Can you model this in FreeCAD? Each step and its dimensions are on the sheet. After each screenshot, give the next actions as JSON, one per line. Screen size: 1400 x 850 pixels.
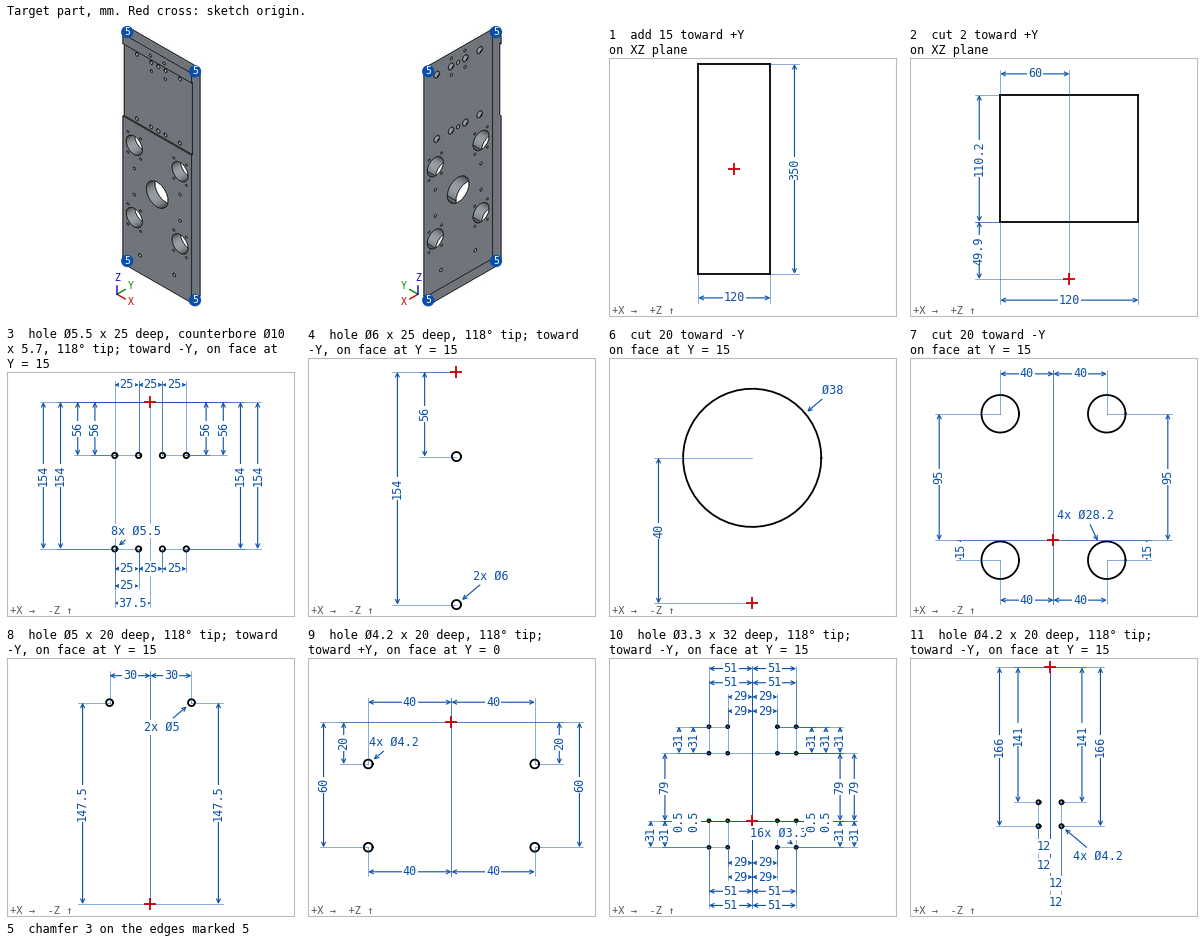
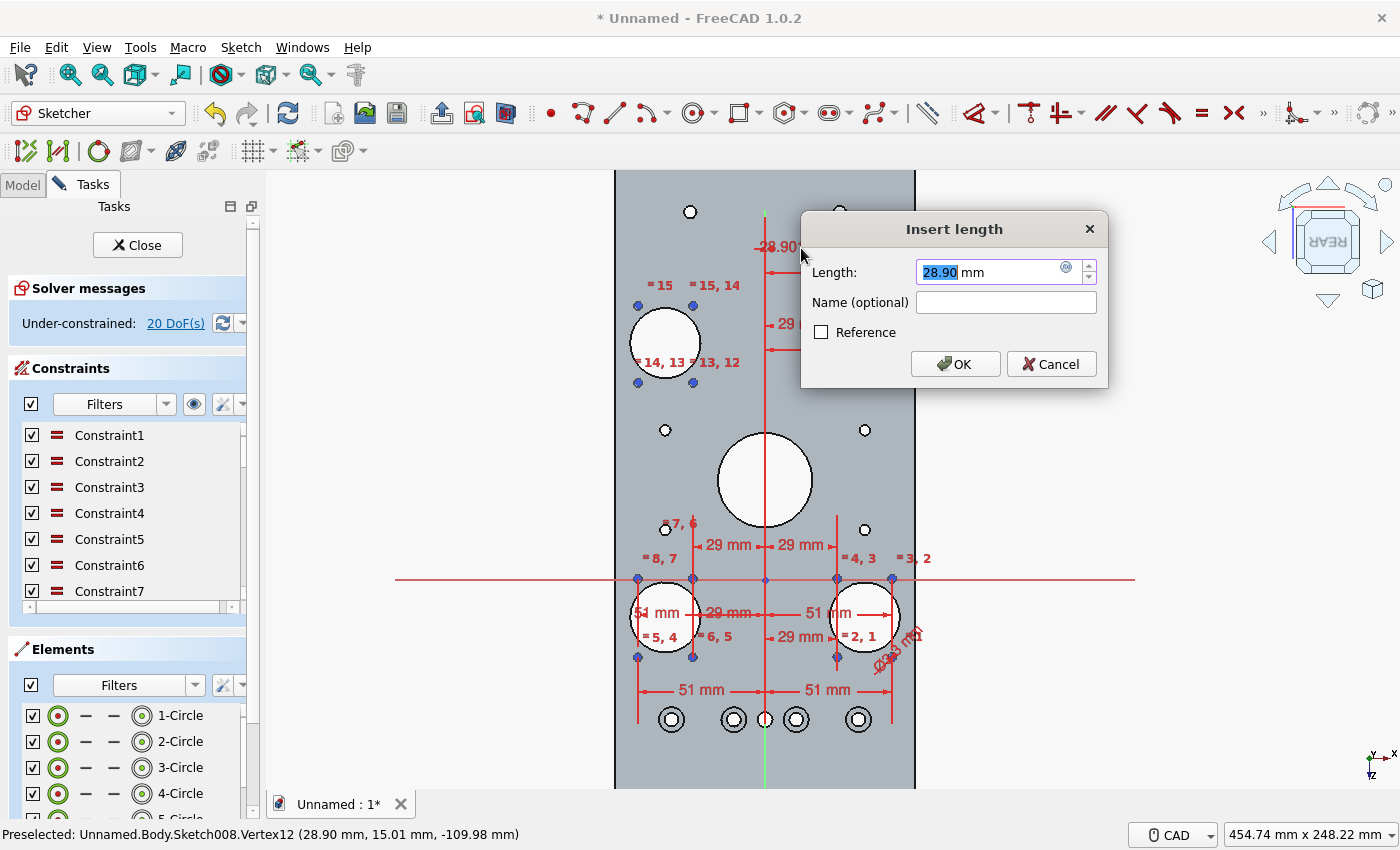
{"action": "type", "text": "29"}
{"action": "key", "text": "Return"}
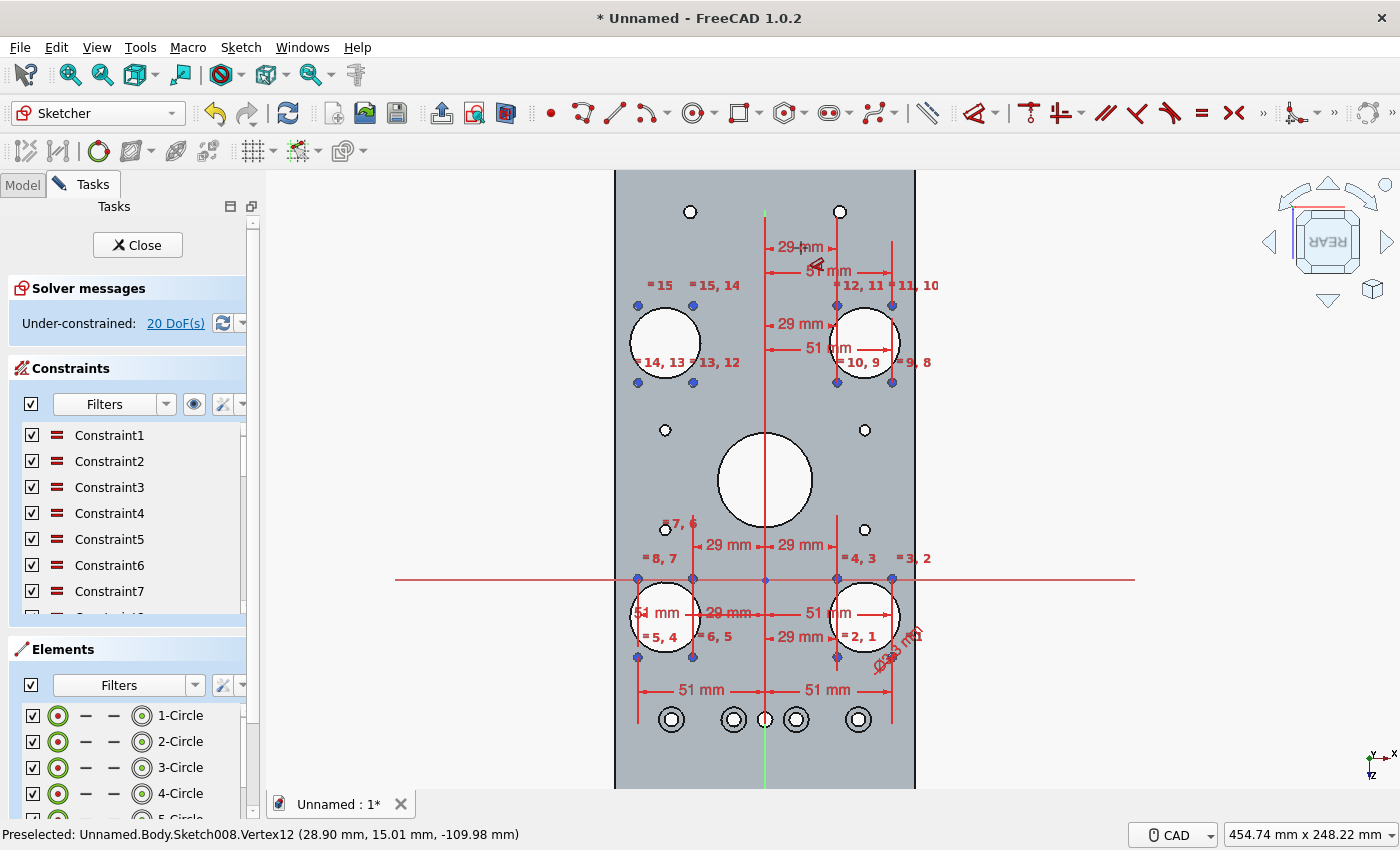
{"action": "left_click", "coordinate": [693, 383]}
{"action": "left_click", "coordinate": [729, 349]}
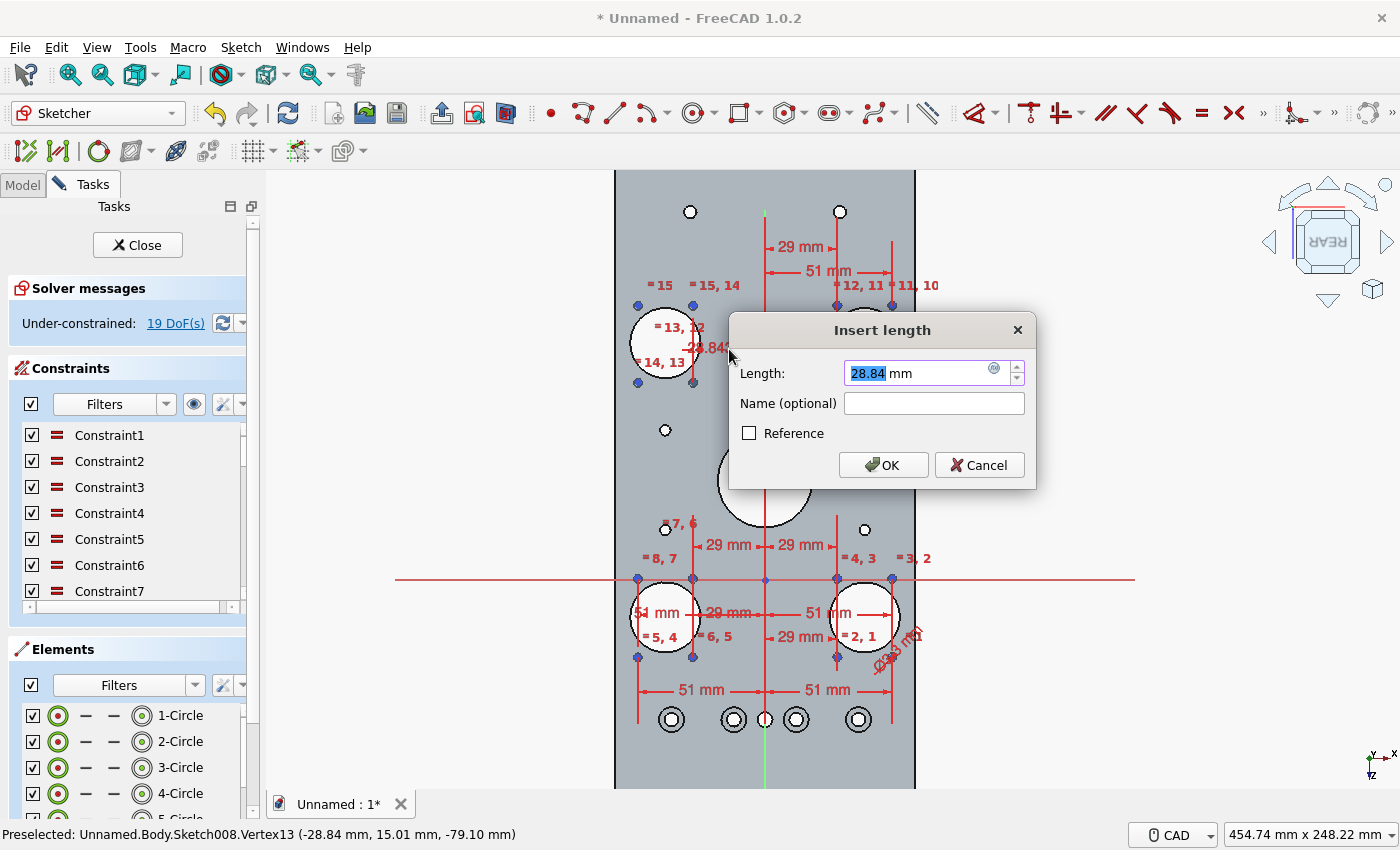
{"action": "type", "text": "29"}
{"action": "key", "text": "Return"}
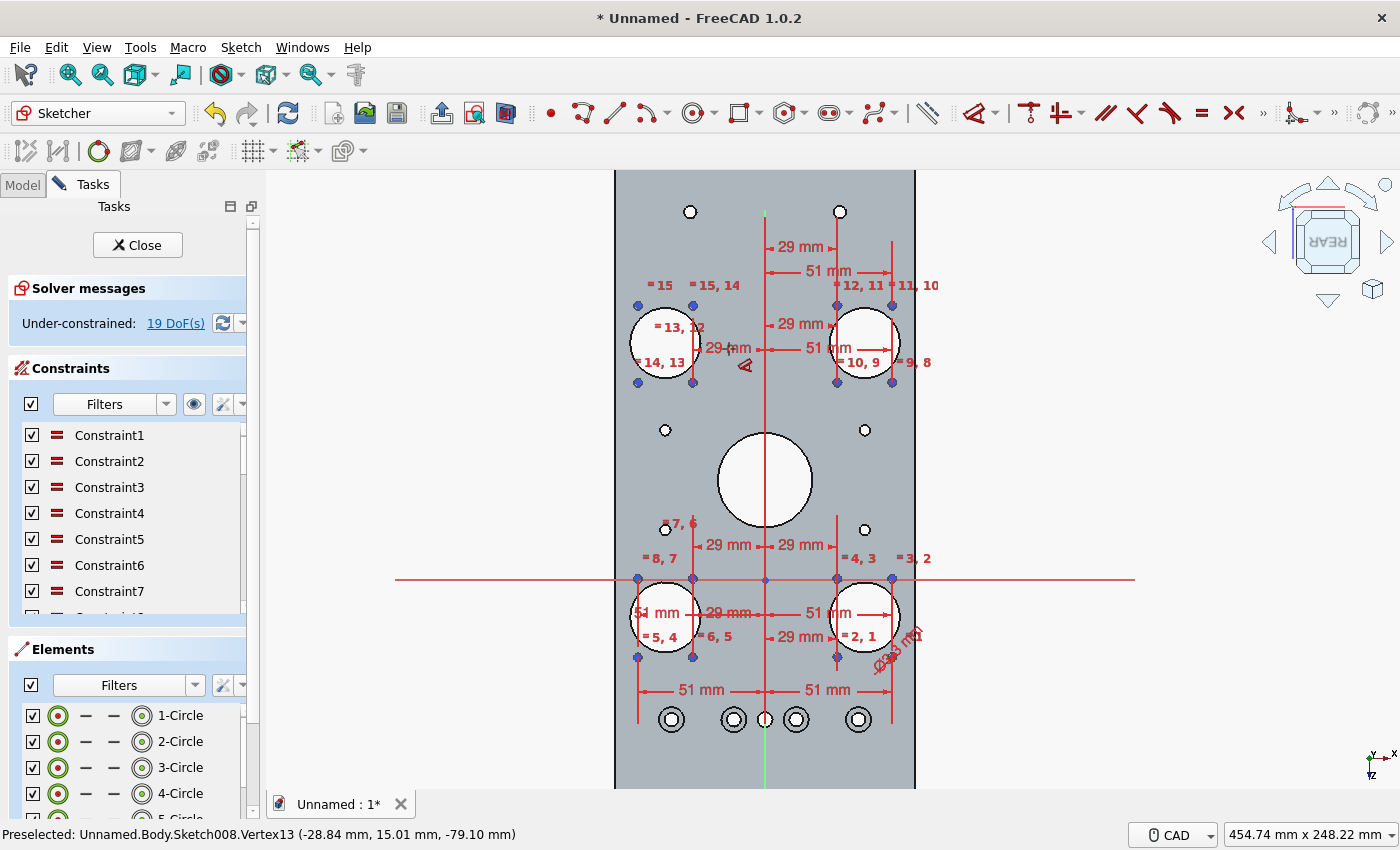
{"action": "left_click", "coordinate": [638, 383]}
{"action": "left_click", "coordinate": [657, 349]}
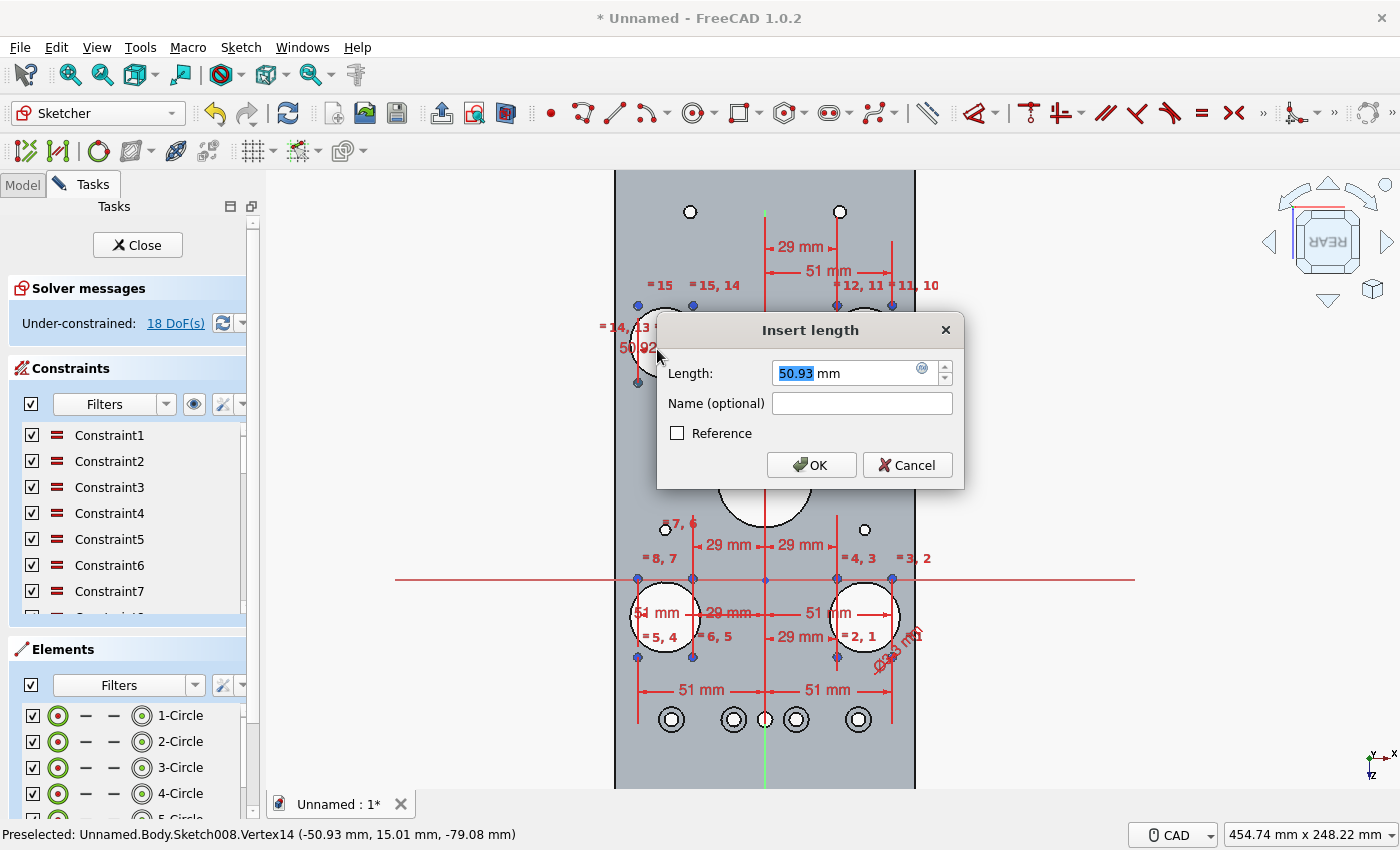
{"action": "type", "text": "51"}
{"action": "key", "text": "Return"}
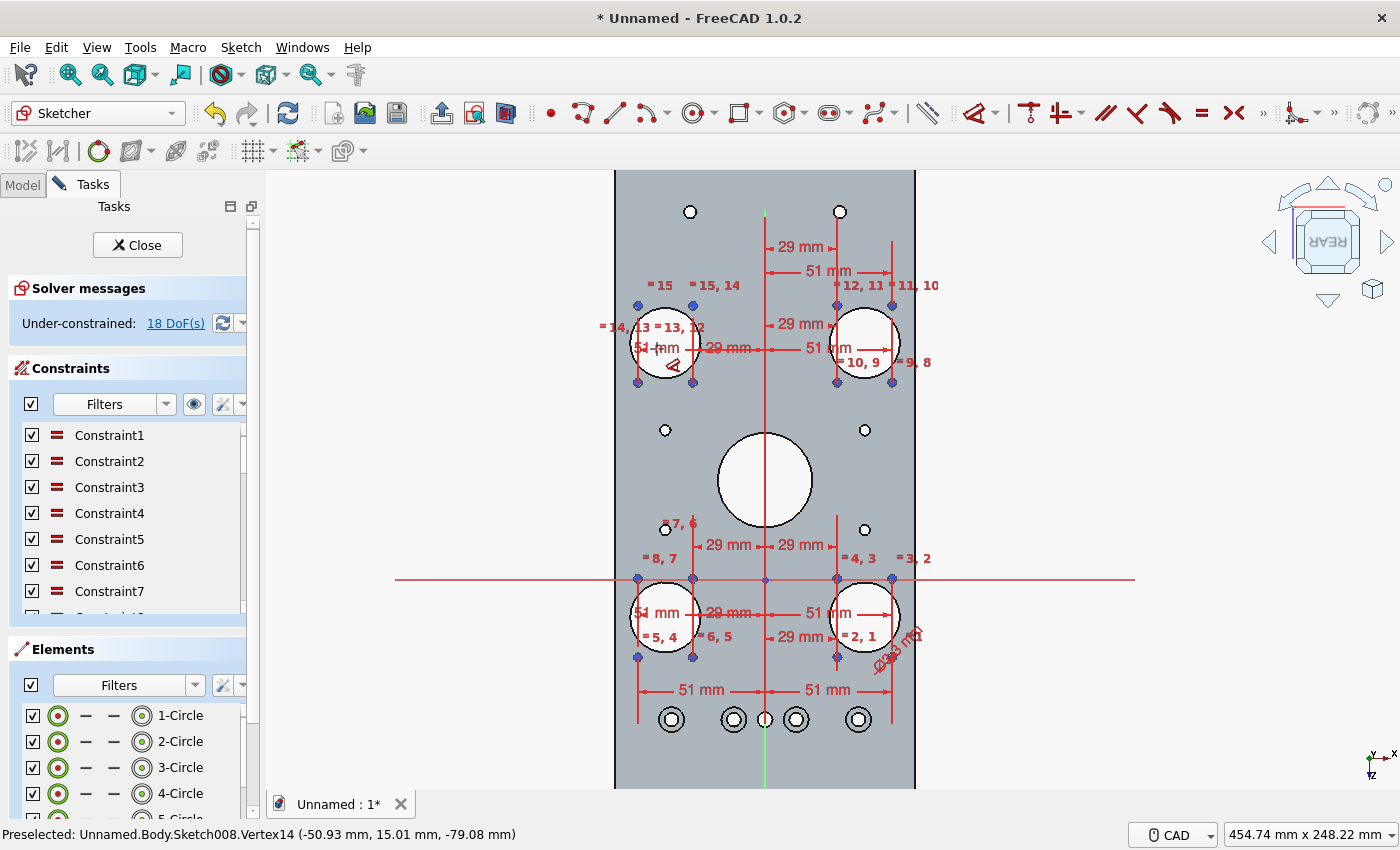
{"action": "left_click", "coordinate": [693, 306]}
{"action": "left_click", "coordinate": [729, 272]}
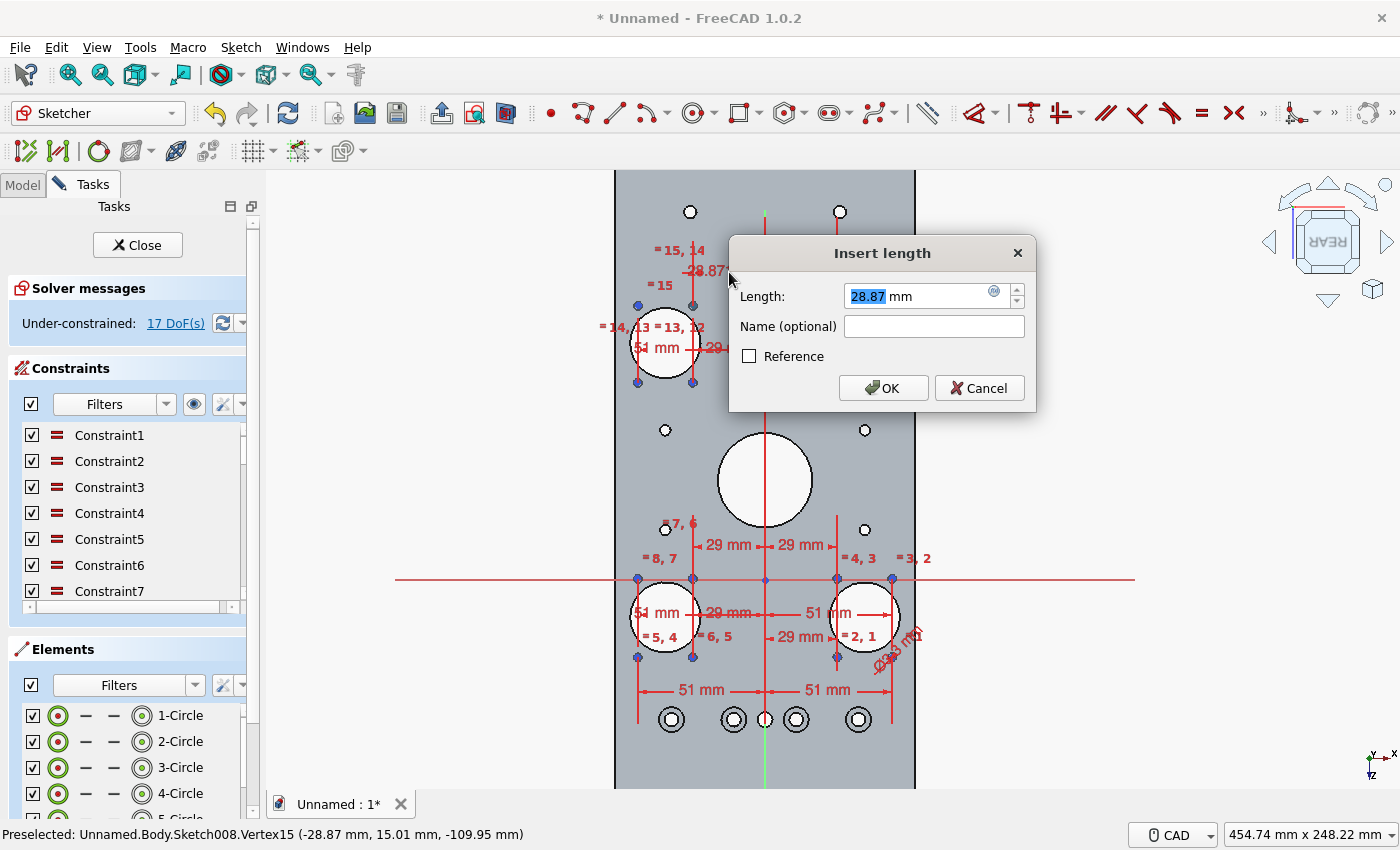
{"action": "type", "text": "29"}
{"action": "key", "text": "Return"}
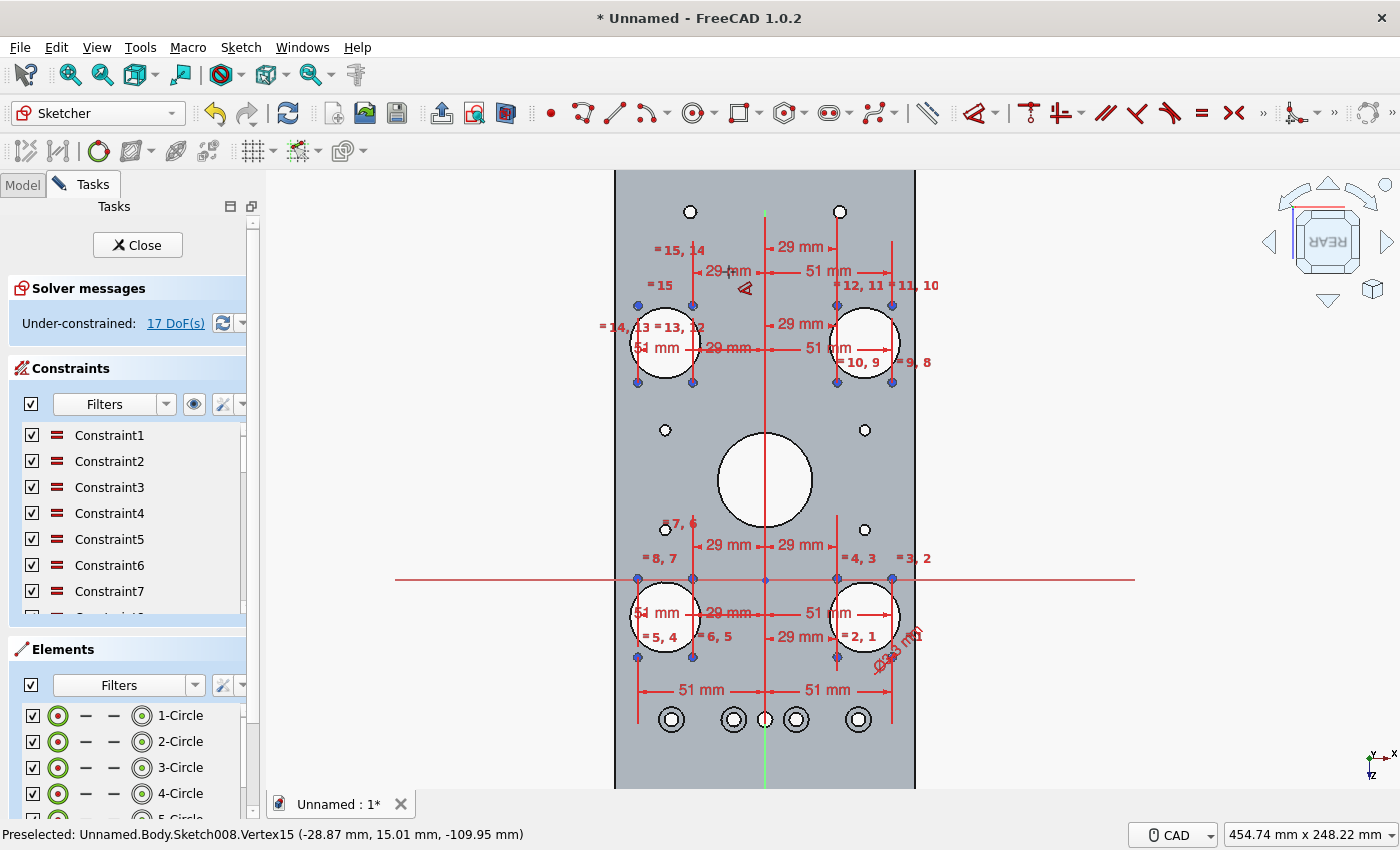
{"action": "left_click", "coordinate": [638, 306]}
{"action": "left_click", "coordinate": [657, 272]}